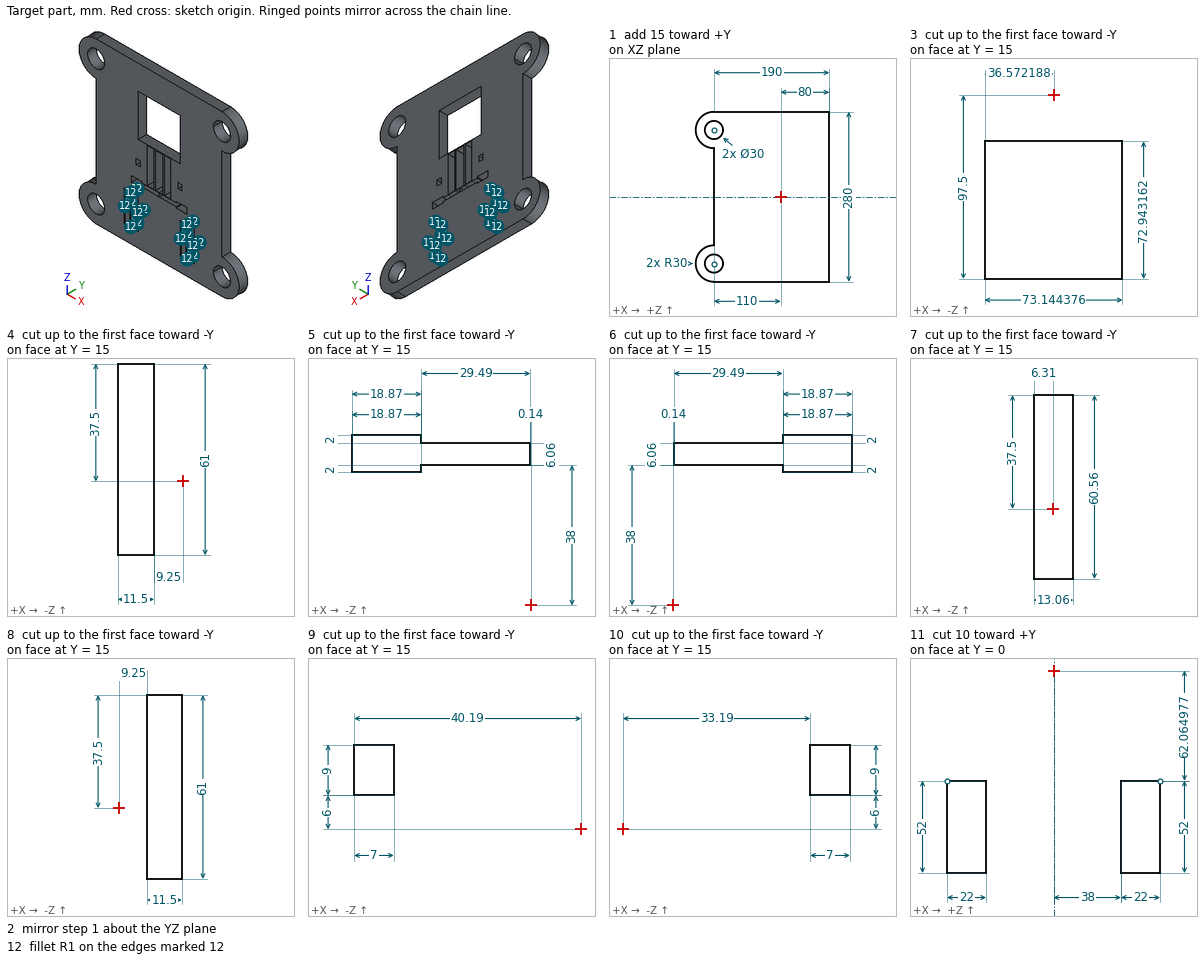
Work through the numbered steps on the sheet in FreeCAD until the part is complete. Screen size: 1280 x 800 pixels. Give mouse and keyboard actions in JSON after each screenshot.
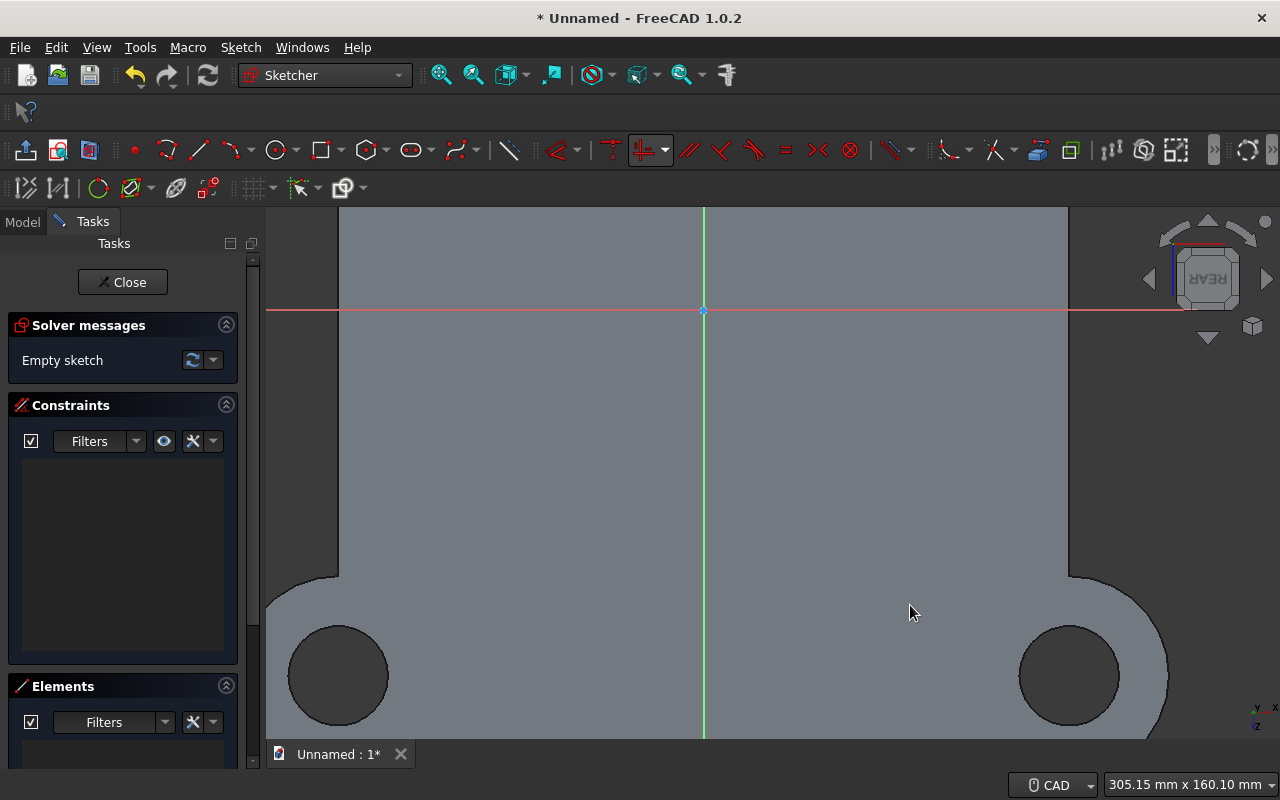
{"action": "key", "text": "g r"}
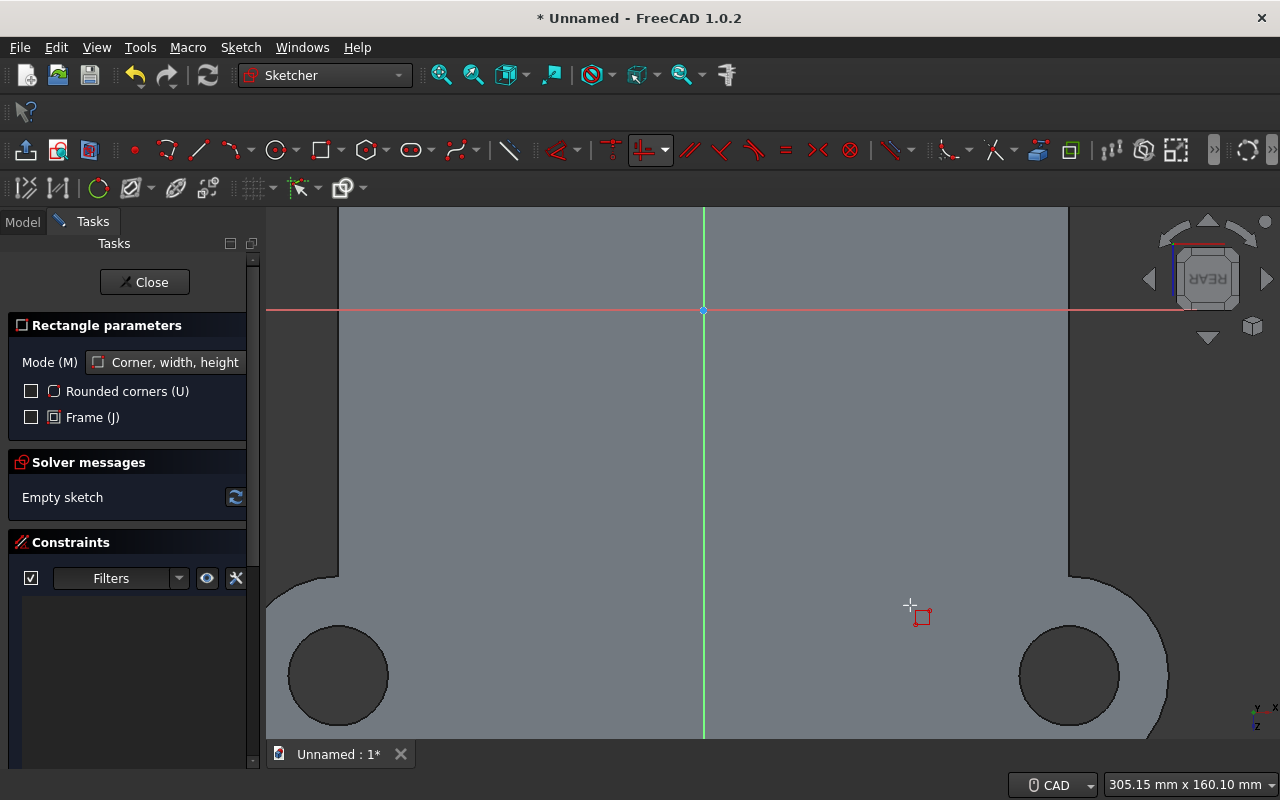
{"action": "left_click", "coordinate": [582, 392]}
{"action": "mouse_move", "coordinate": [825, 634]}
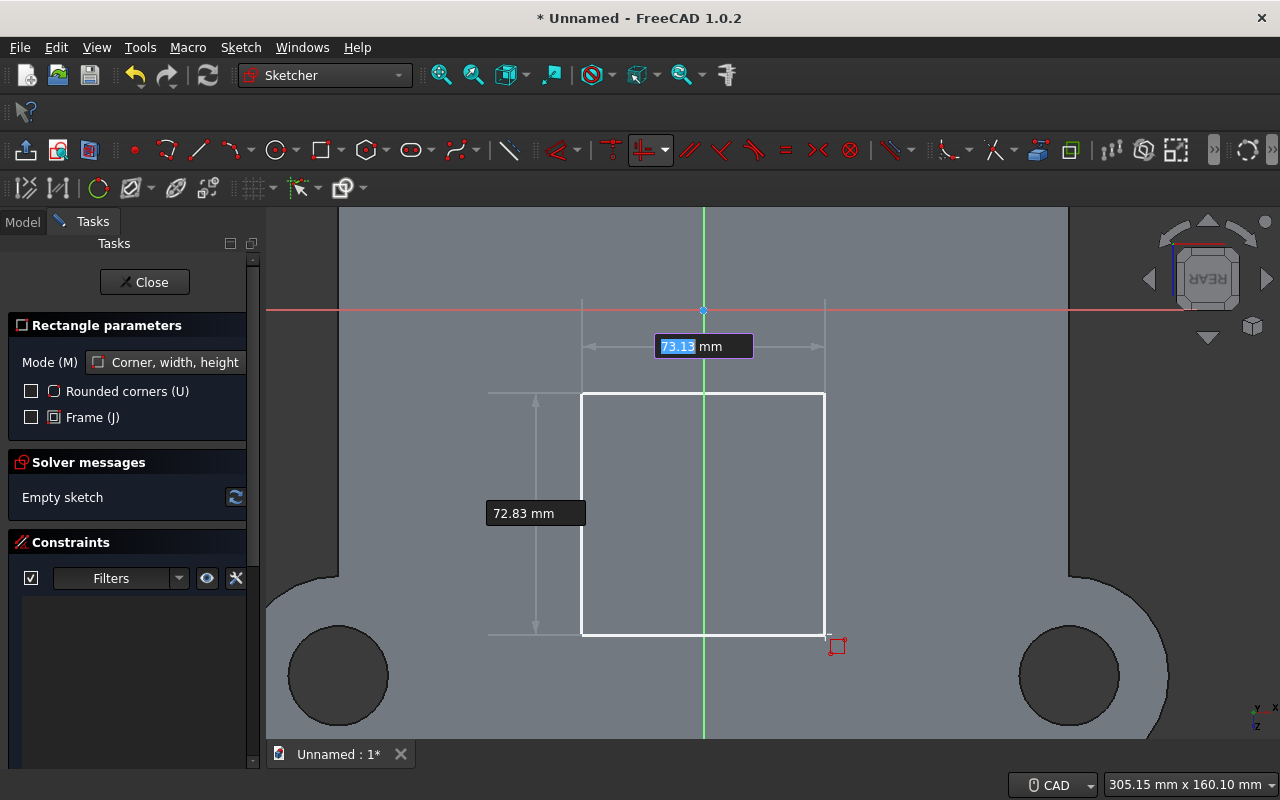
{"action": "type", "text": "73.144376"}
{"action": "key", "text": "Tab"}
{"action": "type", "text": "72.943162"}
{"action": "key", "text": "Return"}
{"action": "key", "text": "Escape"}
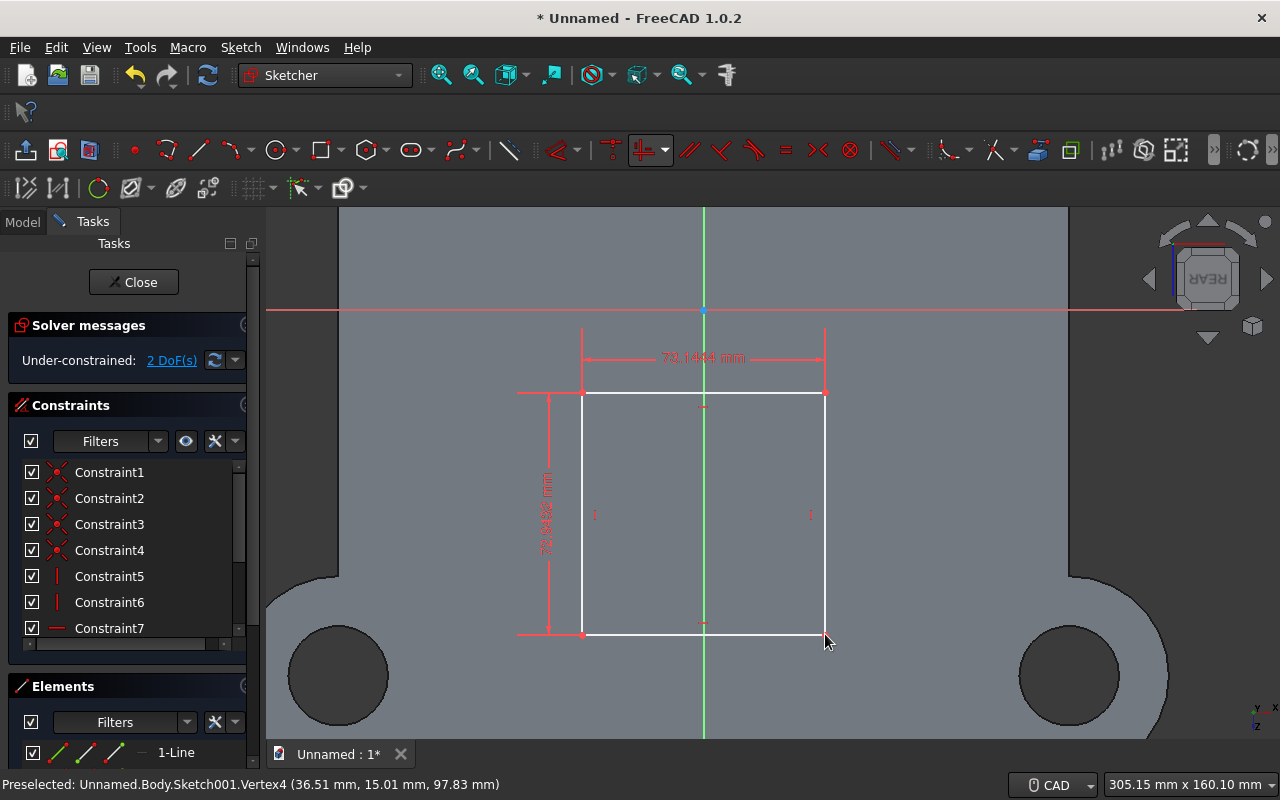
{"action": "left_click", "coordinate": [556, 150]}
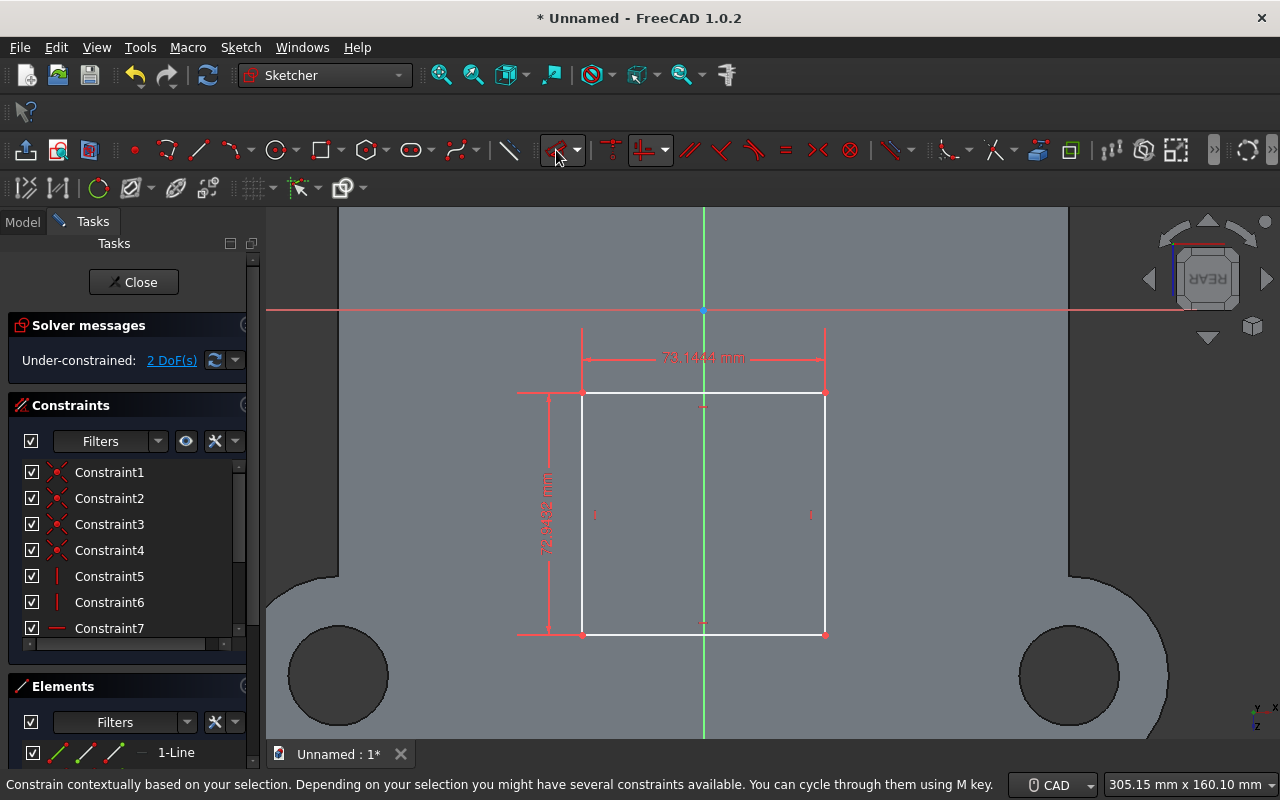
{"action": "left_click", "coordinate": [582, 635]}
{"action": "left_click", "coordinate": [548, 473]}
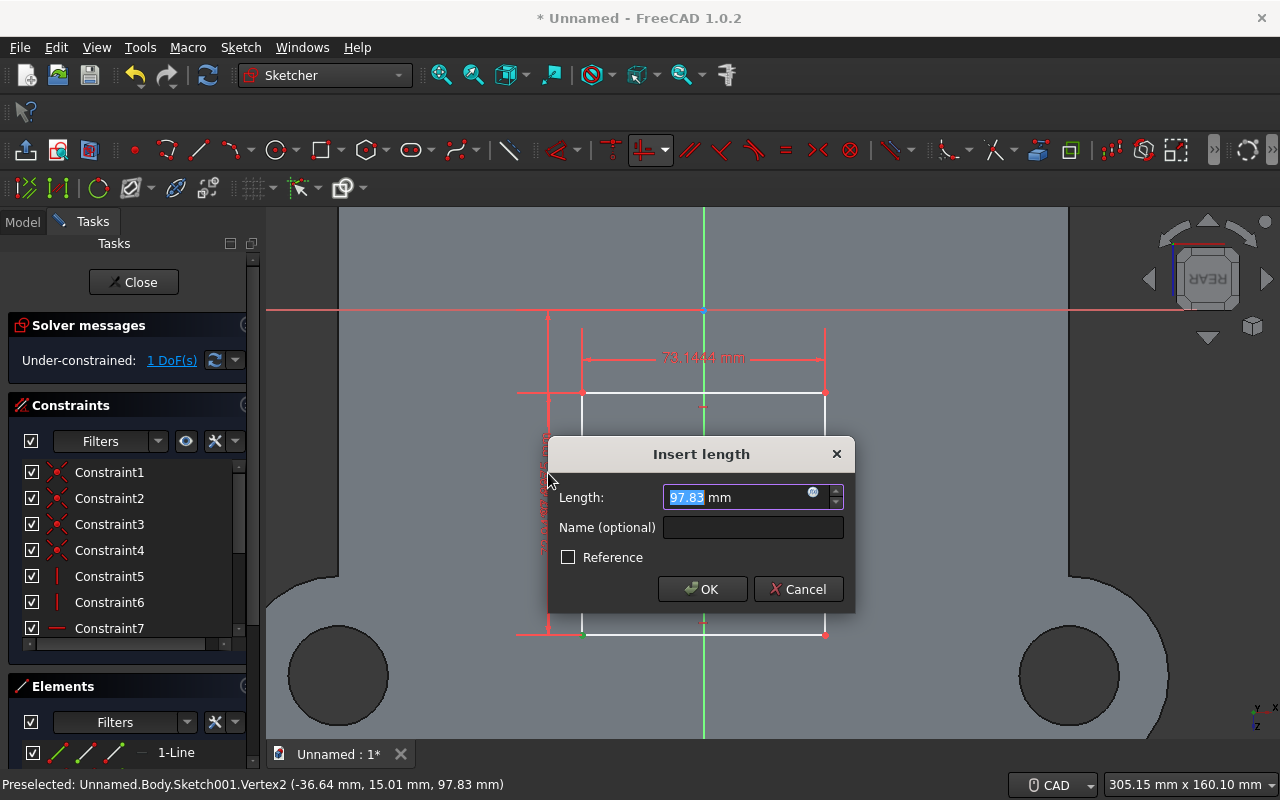
{"action": "type", "text": "97.5"}
{"action": "key", "text": "Return"}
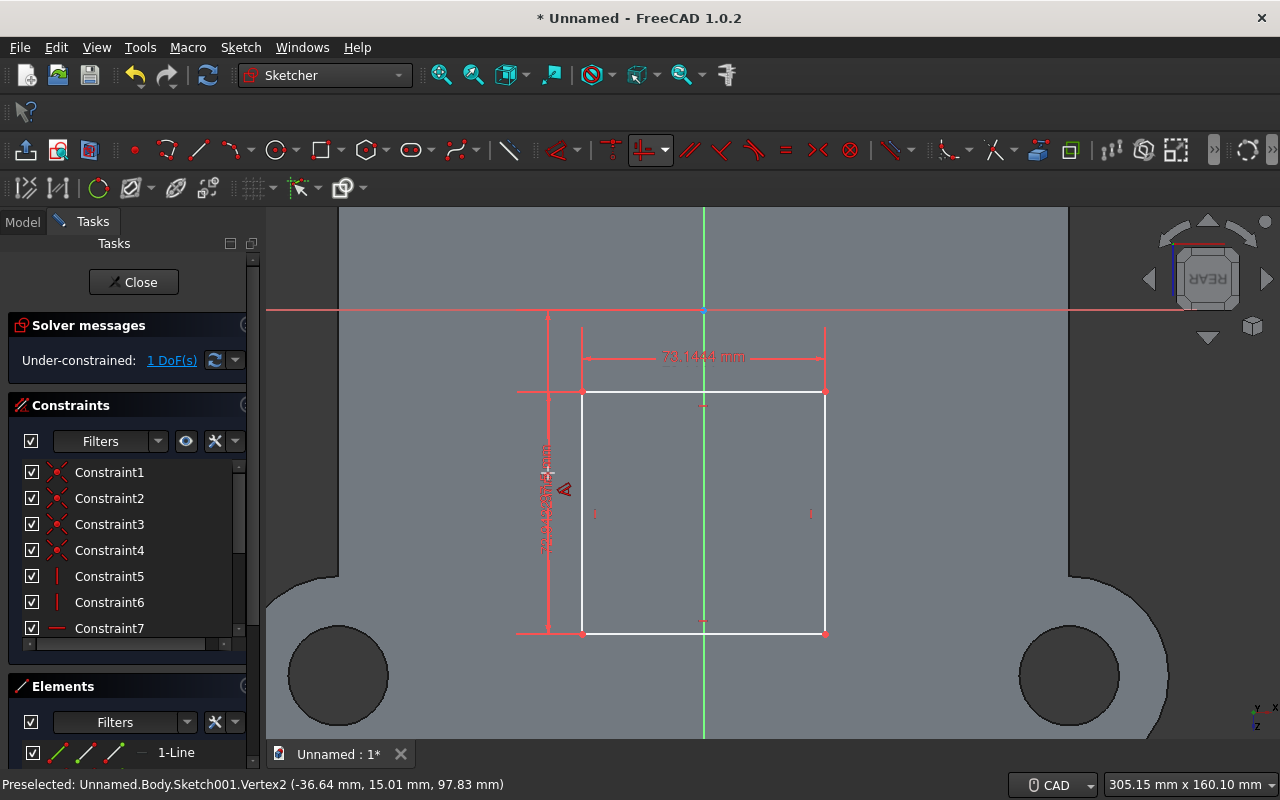
{"action": "left_click", "coordinate": [582, 392]}
{"action": "left_click", "coordinate": [643, 276]}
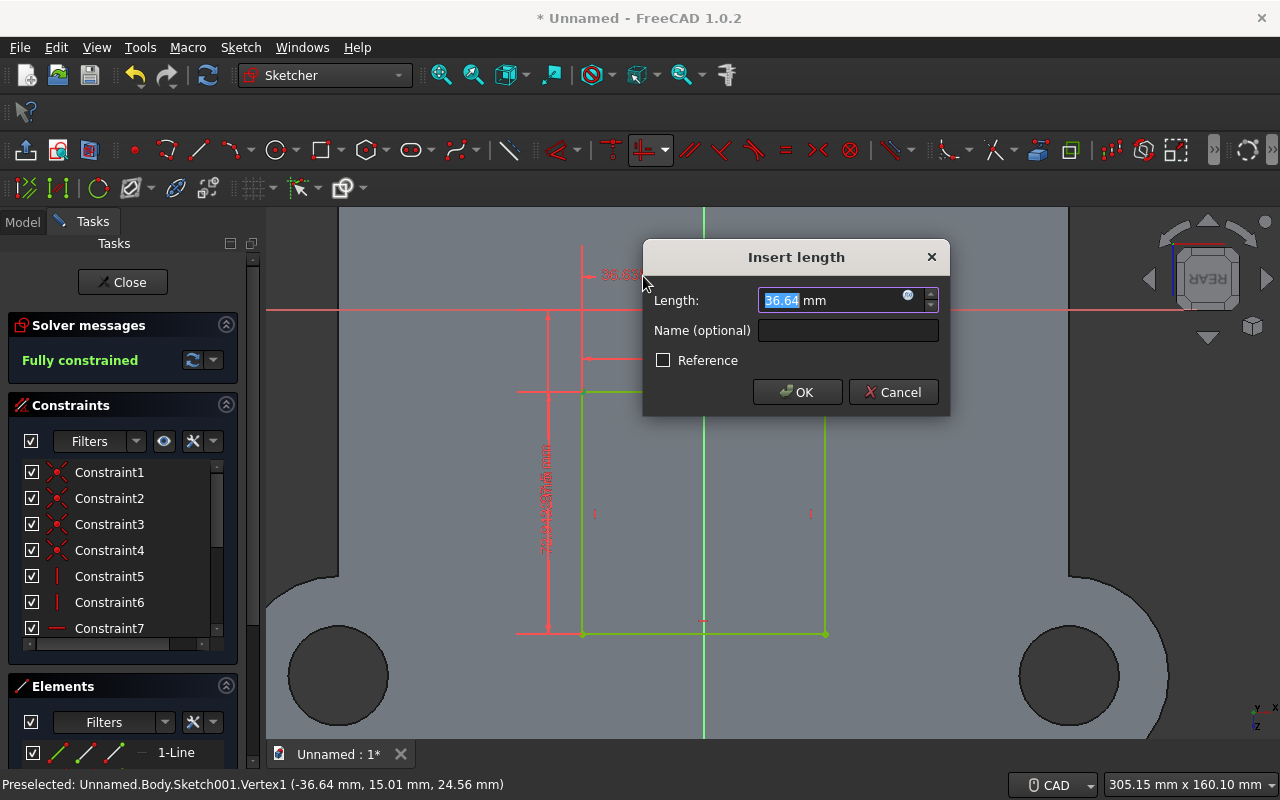
{"action": "type", "text": "36.572188"}
{"action": "key", "text": "Return"}
{"action": "key", "text": "Escape"}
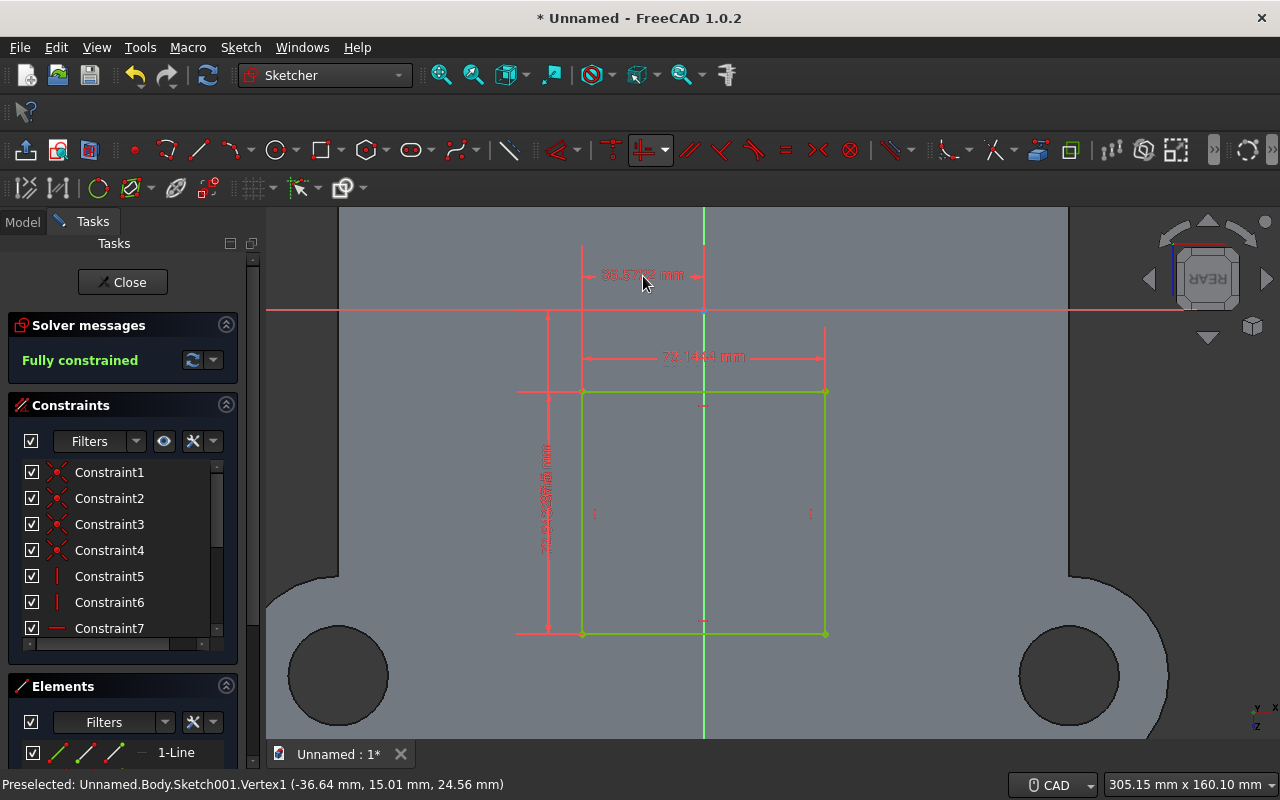
{"action": "left_click", "coordinate": [123, 282]}